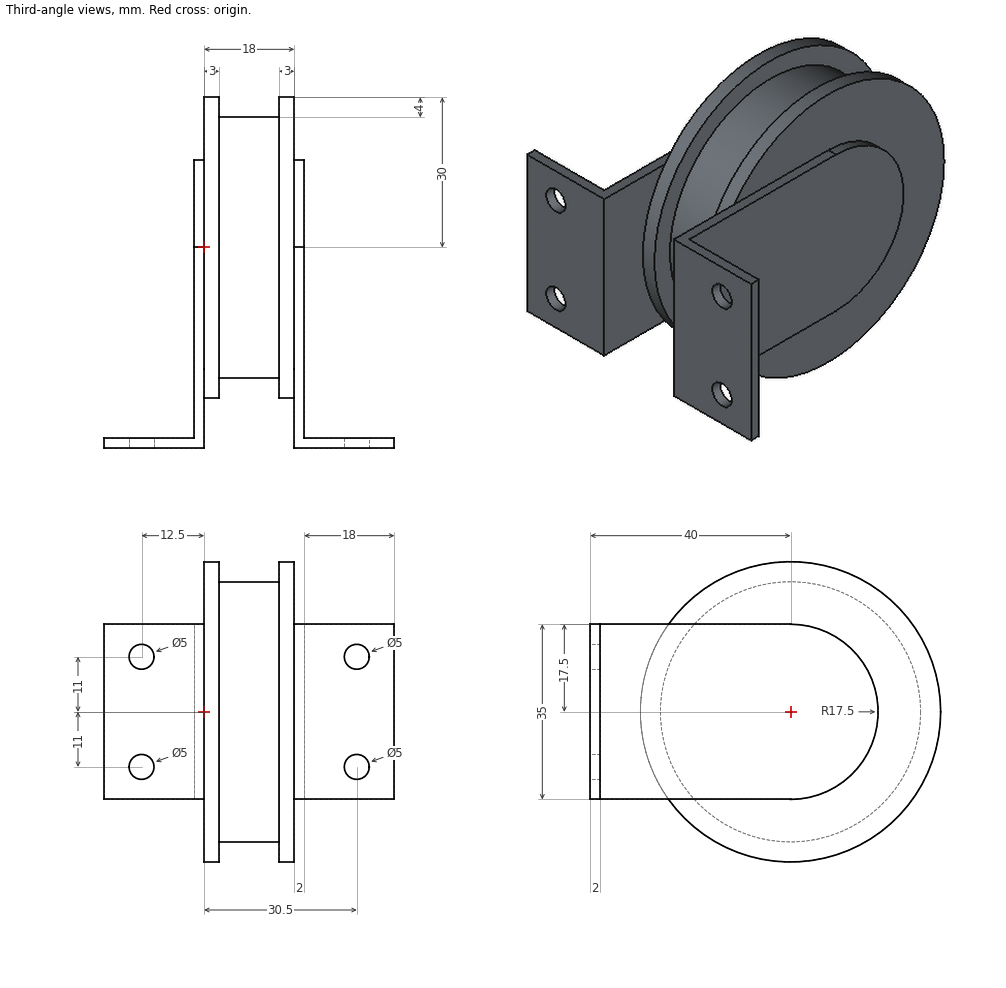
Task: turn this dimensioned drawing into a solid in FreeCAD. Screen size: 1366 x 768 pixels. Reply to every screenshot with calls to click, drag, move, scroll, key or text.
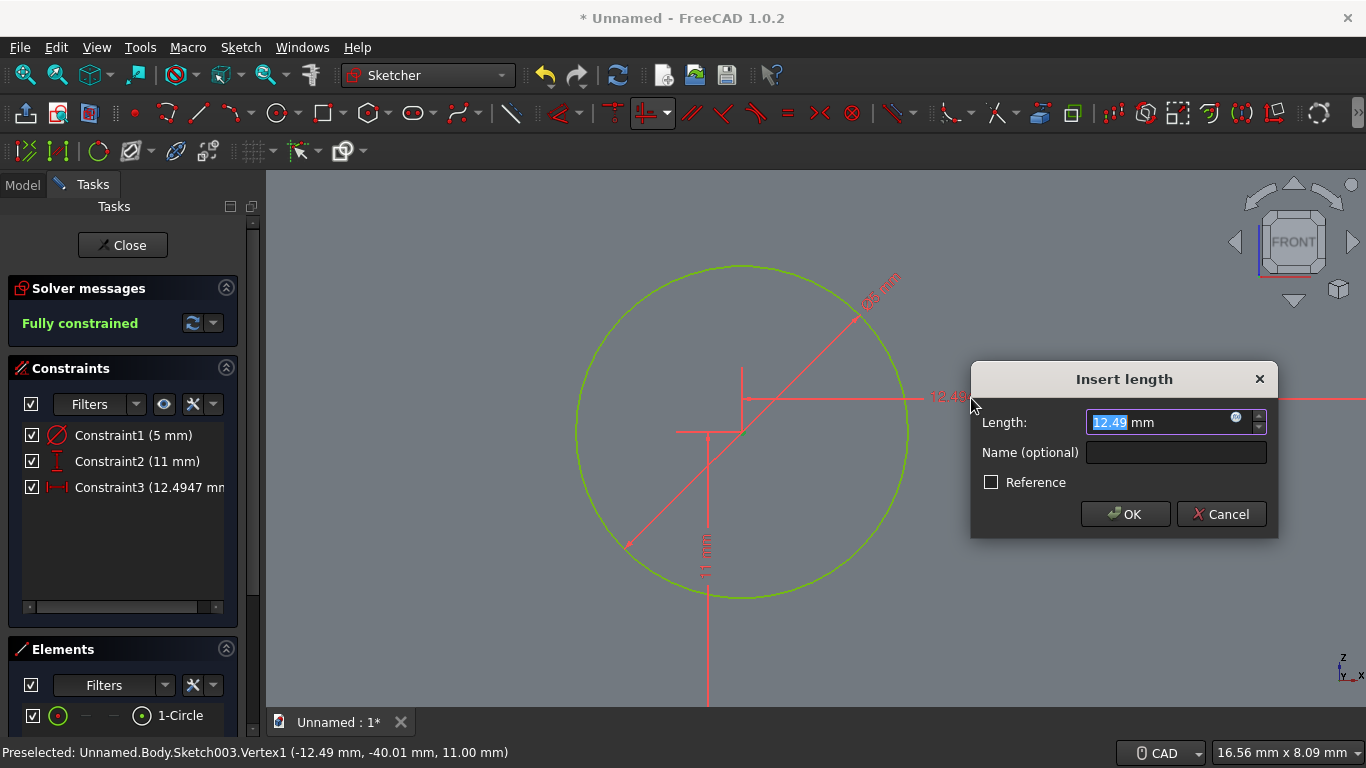
text(12.5)
key(Return)
key(Escape)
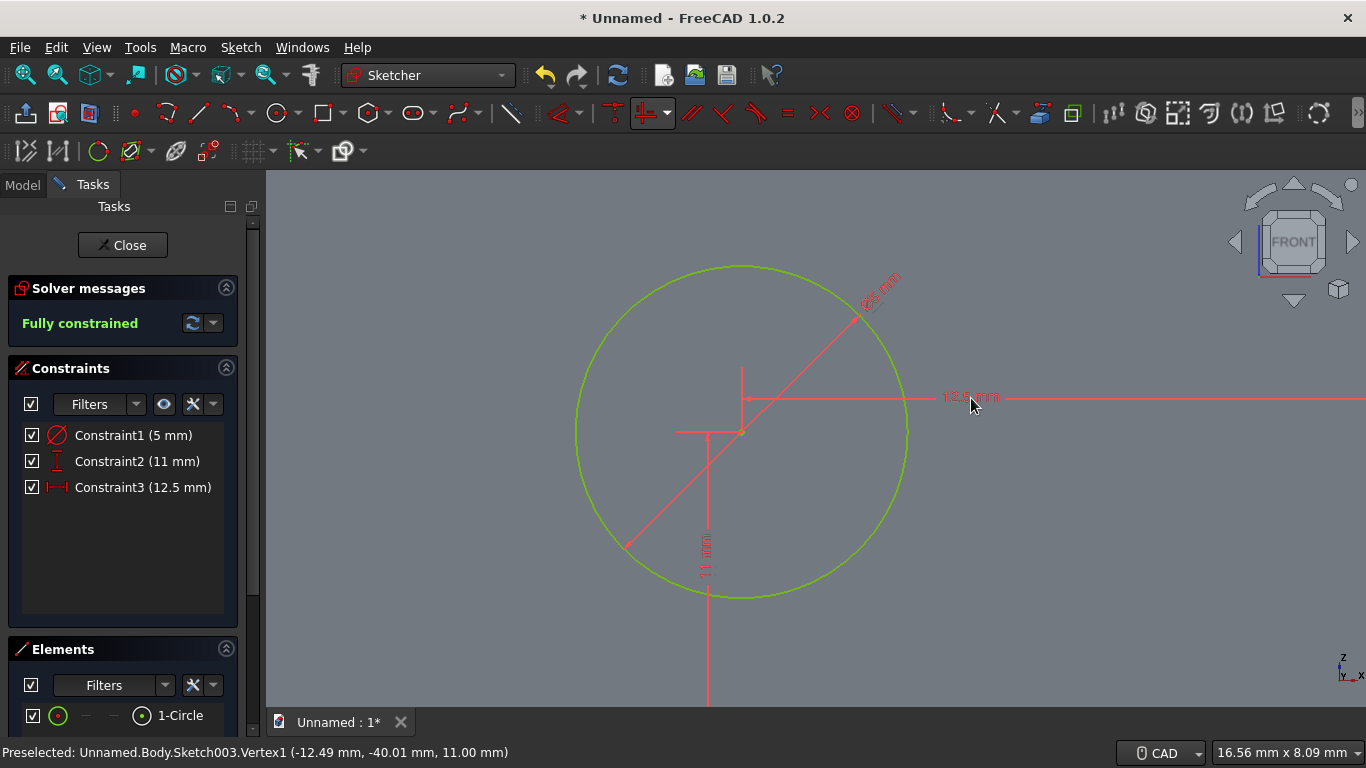
click(123, 245)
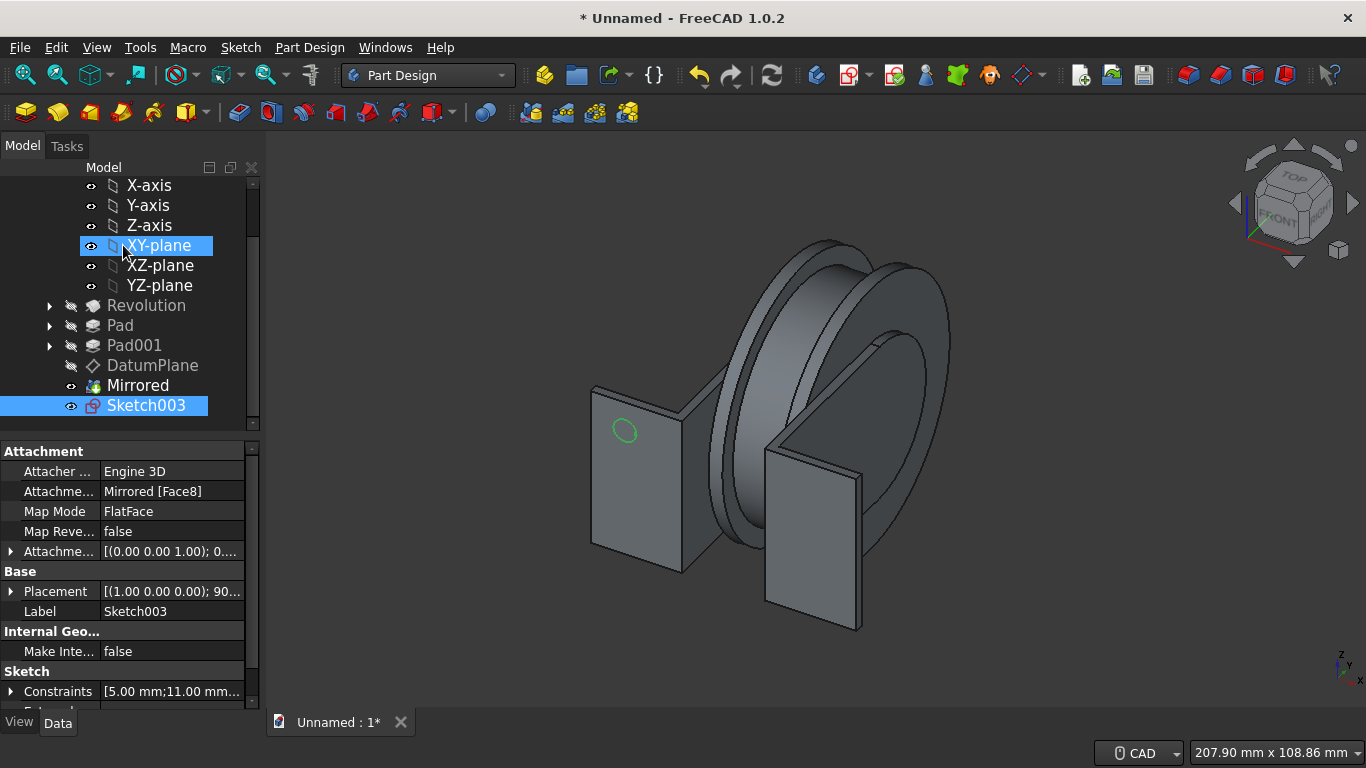
click(240, 112)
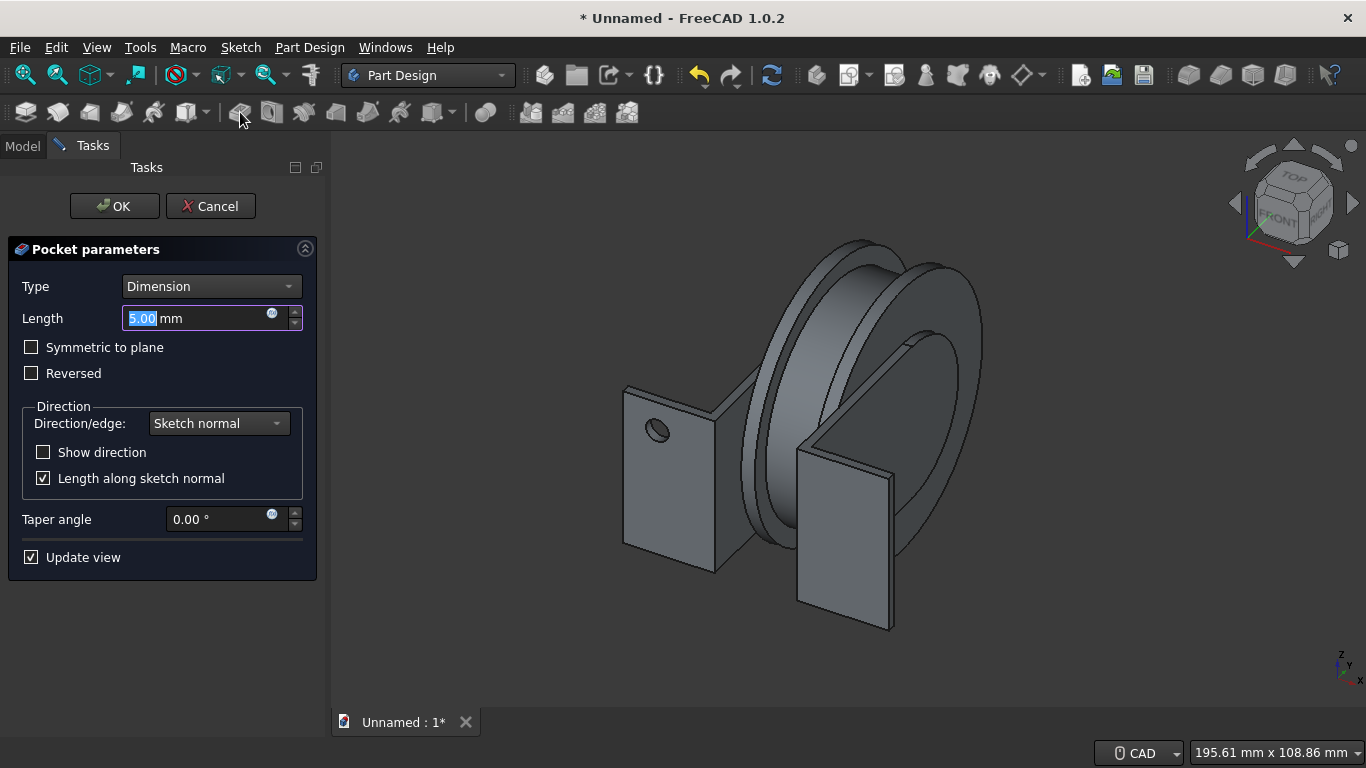
click(212, 286)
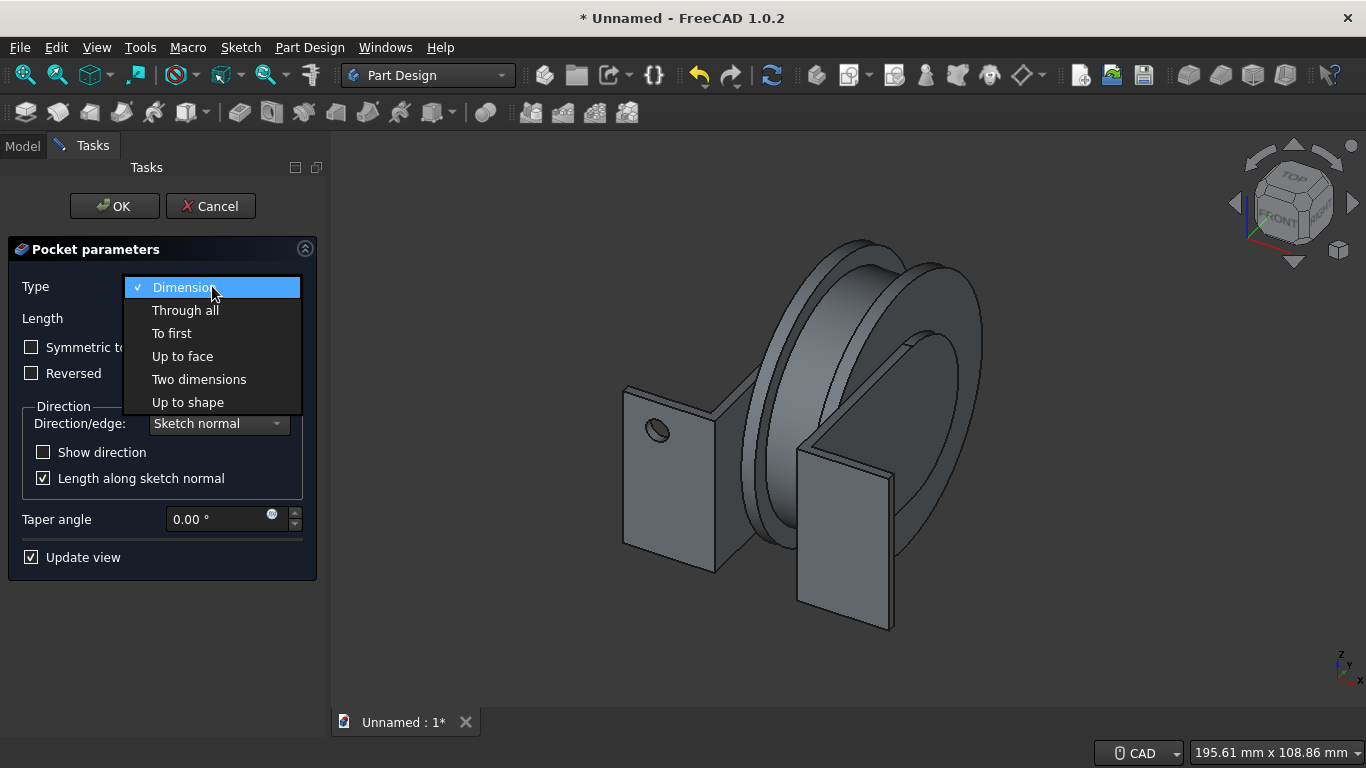
click(212, 334)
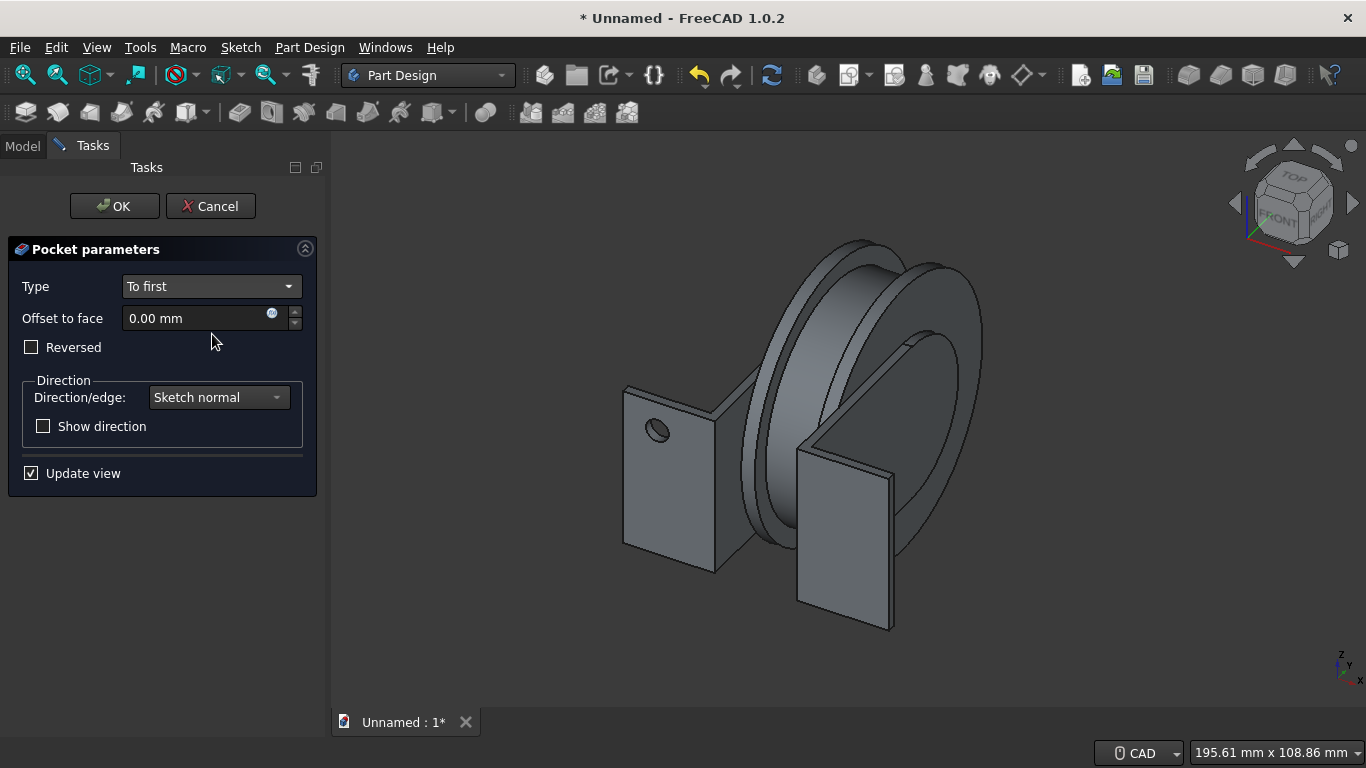
click(115, 206)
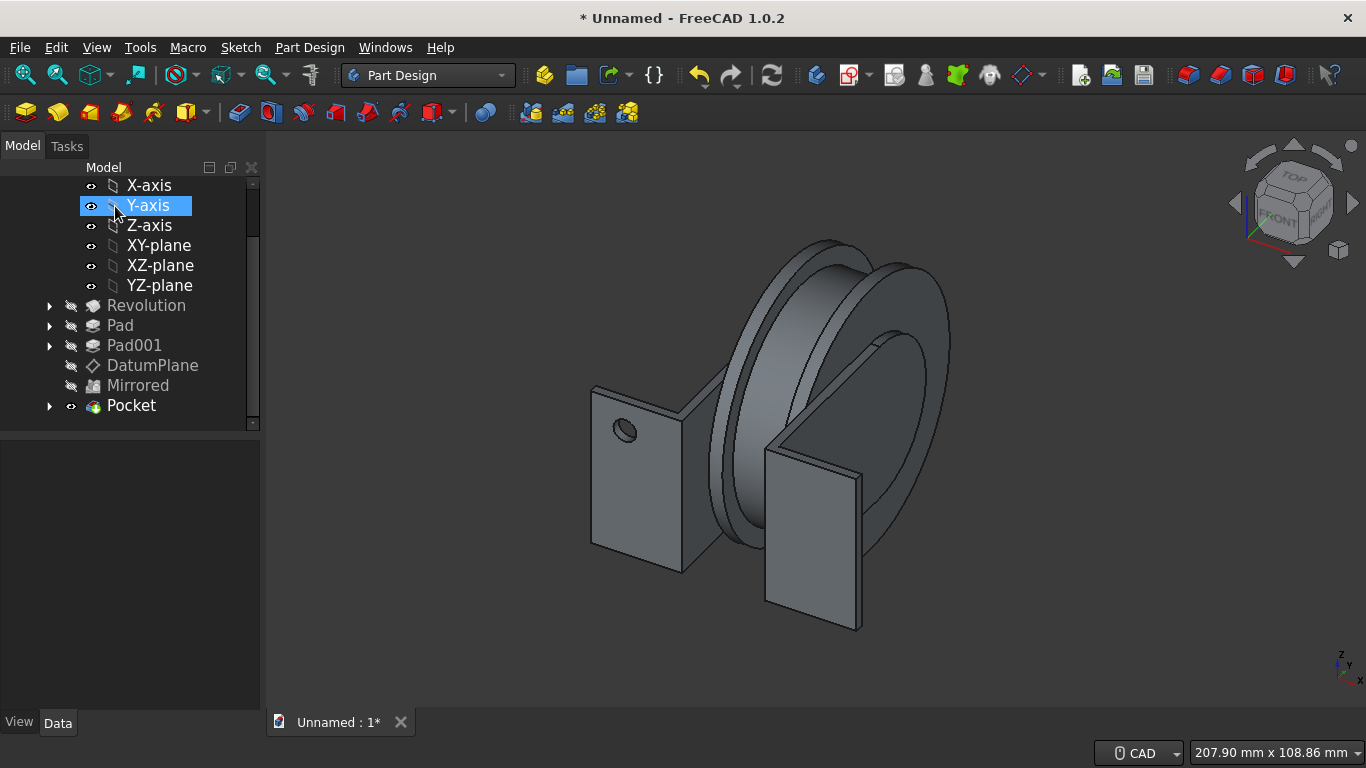
click(810, 517)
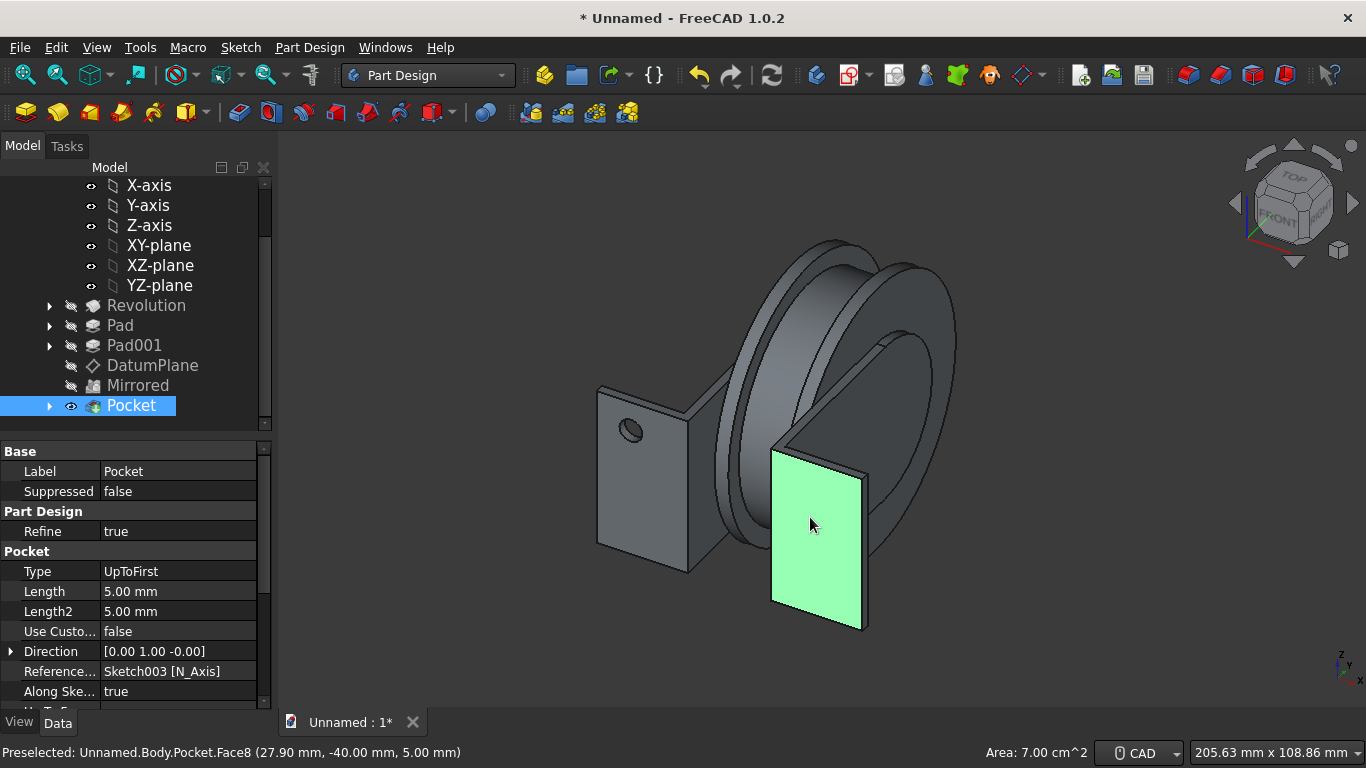
click(850, 76)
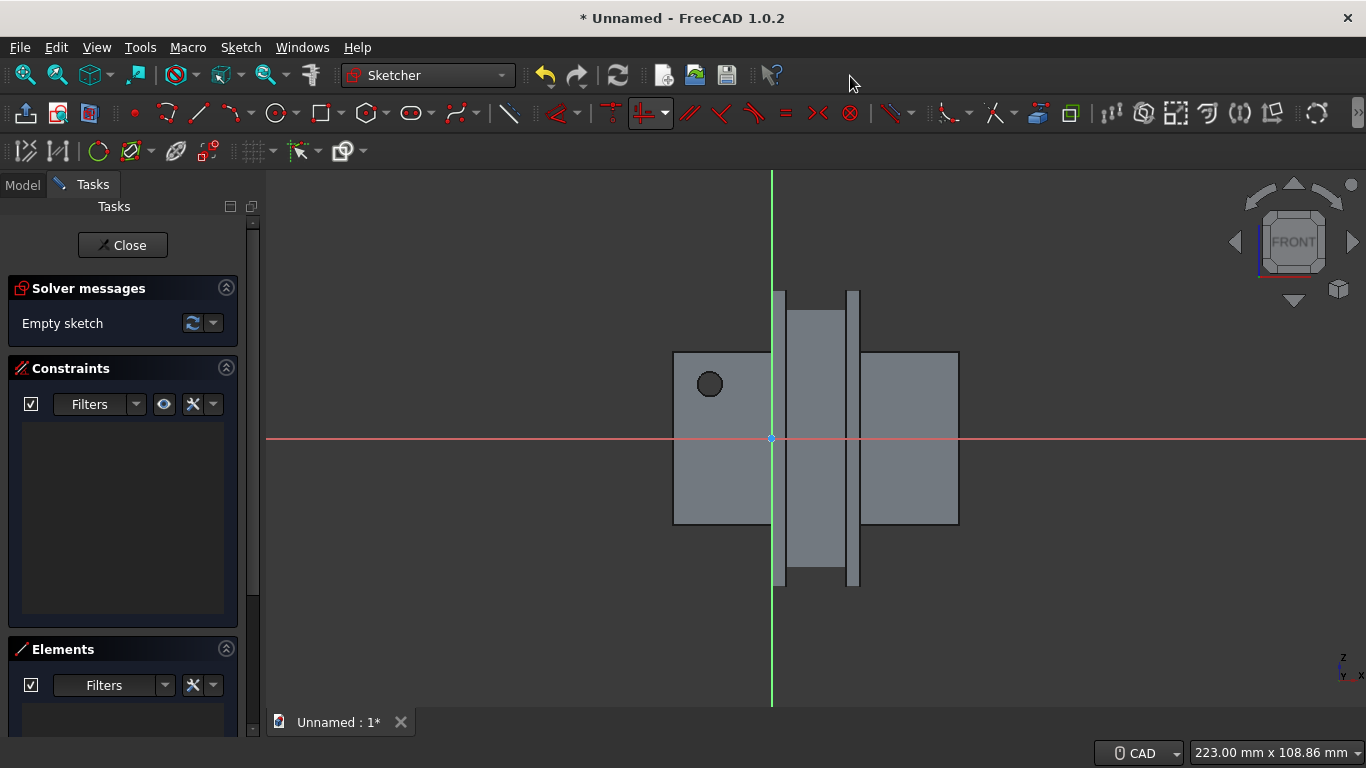
scroll(707, 497, up, 13)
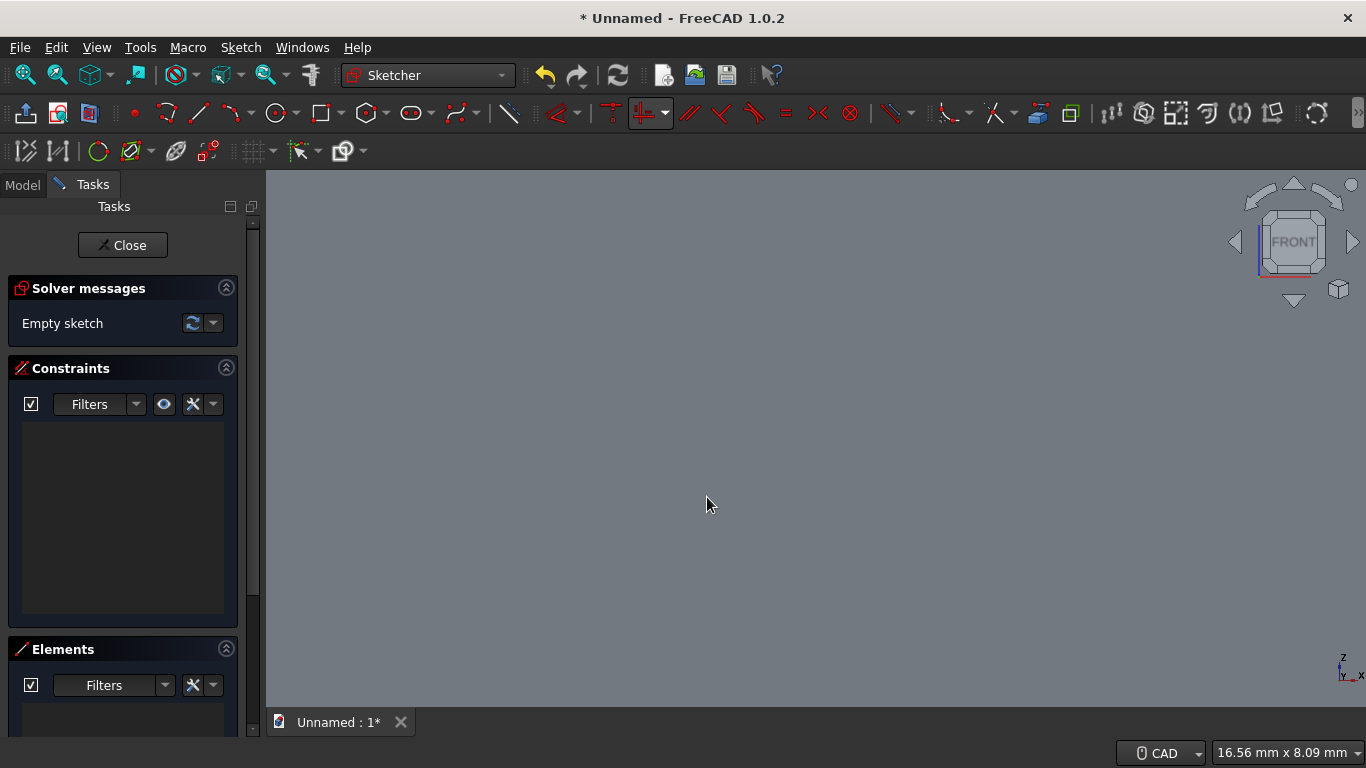
click(276, 114)